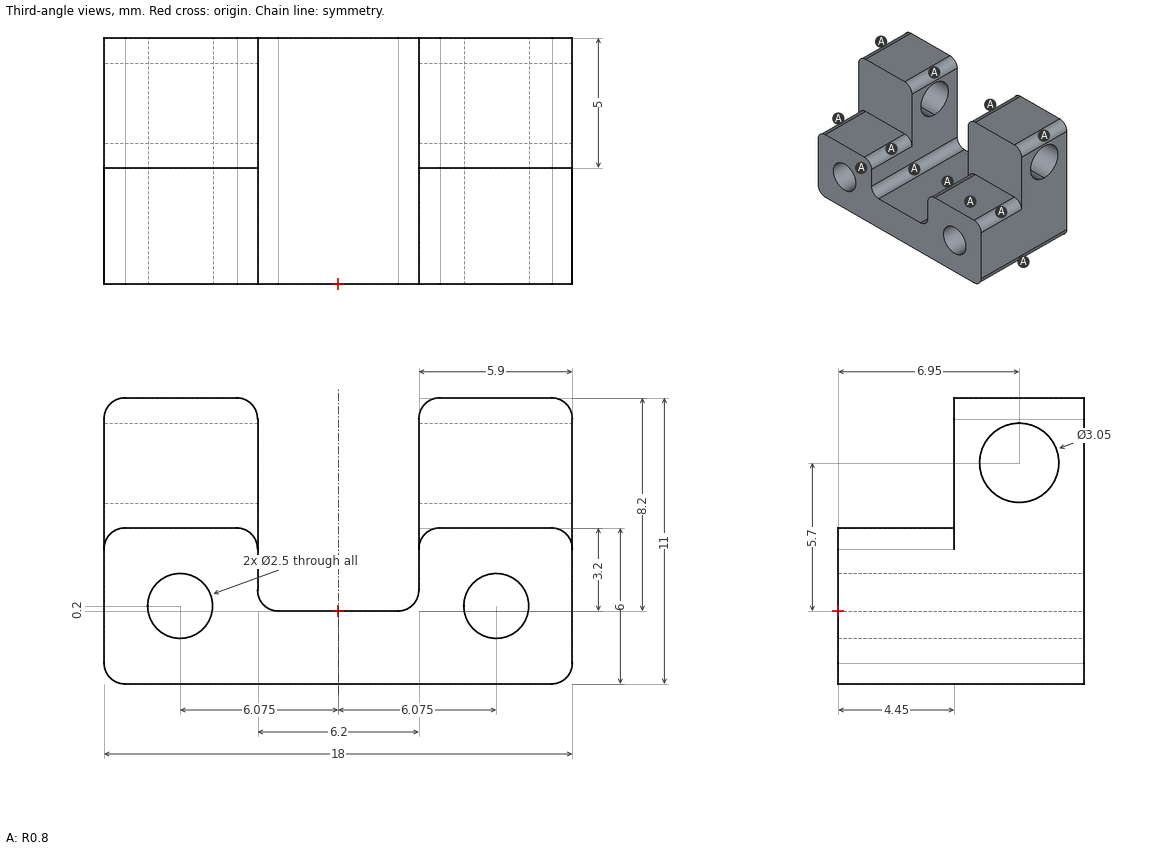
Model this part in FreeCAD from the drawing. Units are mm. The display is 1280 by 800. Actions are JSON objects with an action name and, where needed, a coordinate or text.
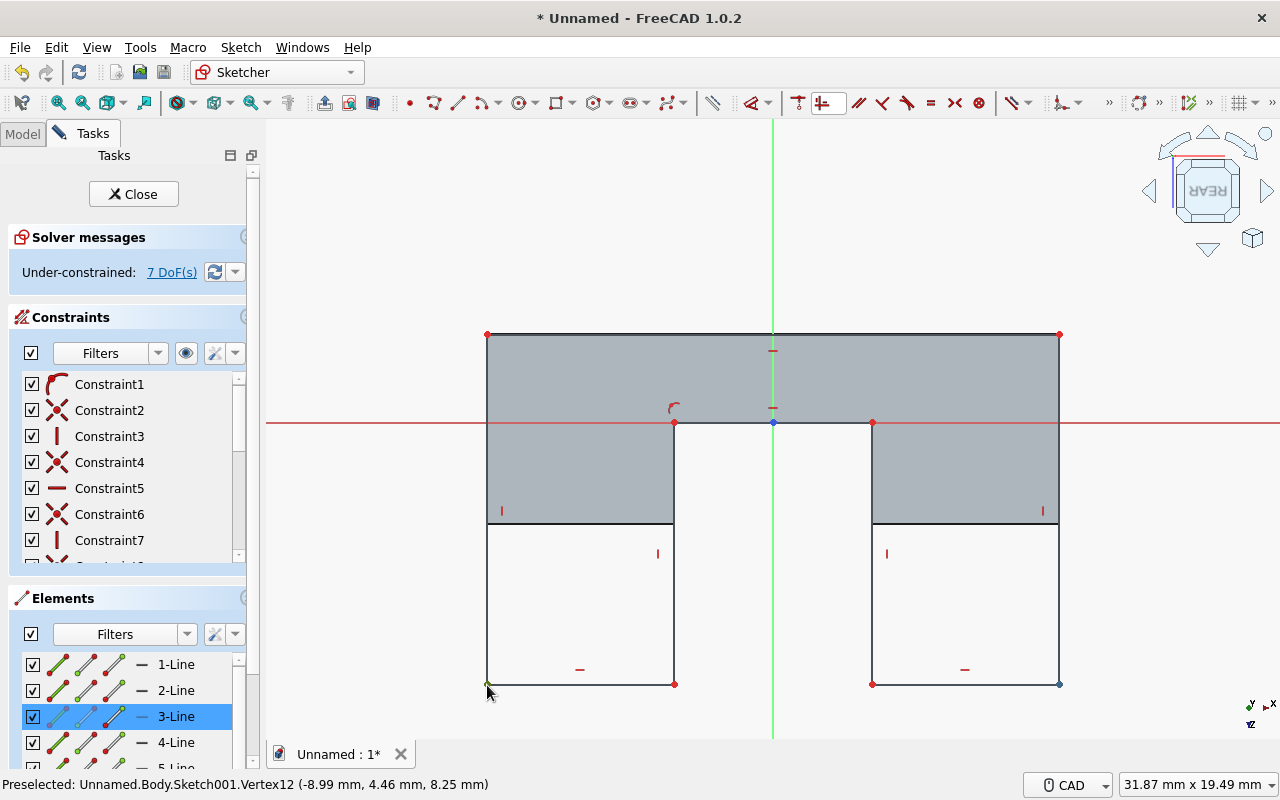
{"action": "left_click", "coordinate": [773, 671]}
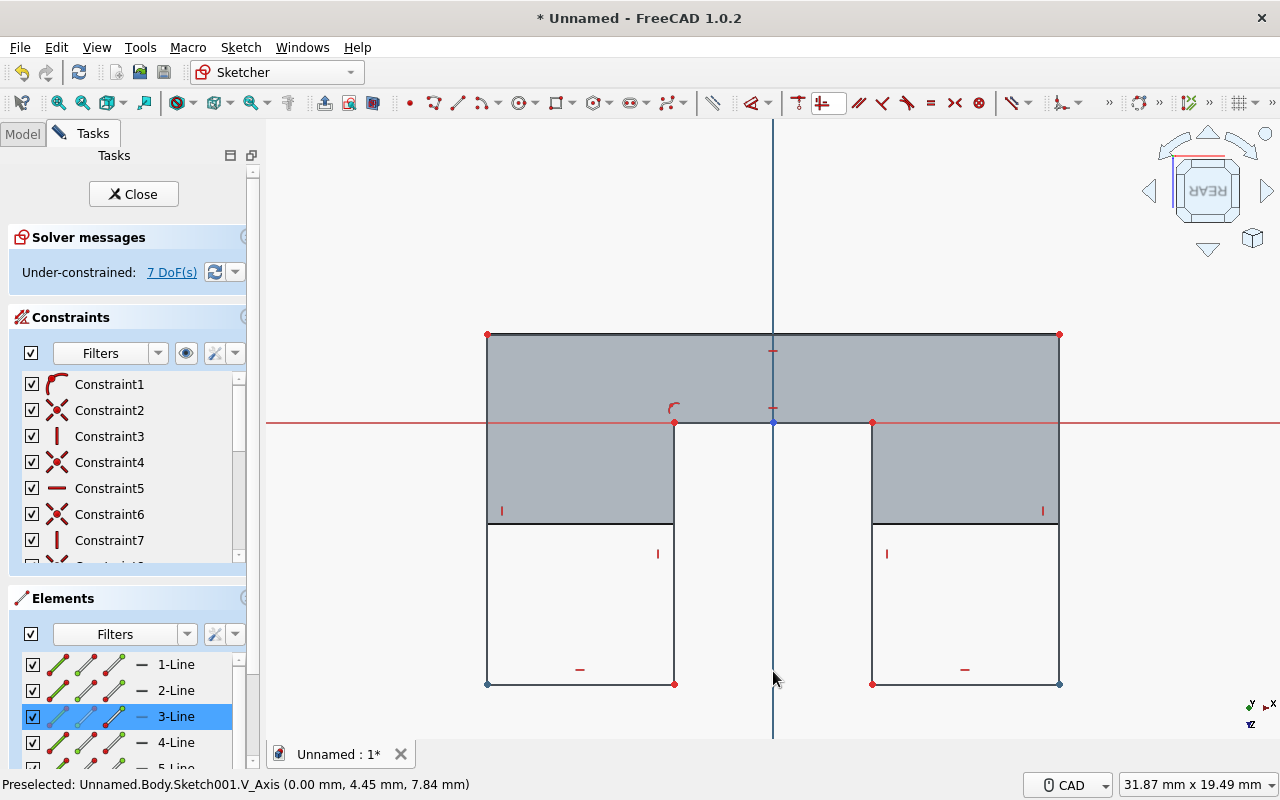
{"action": "left_click", "coordinate": [956, 104]}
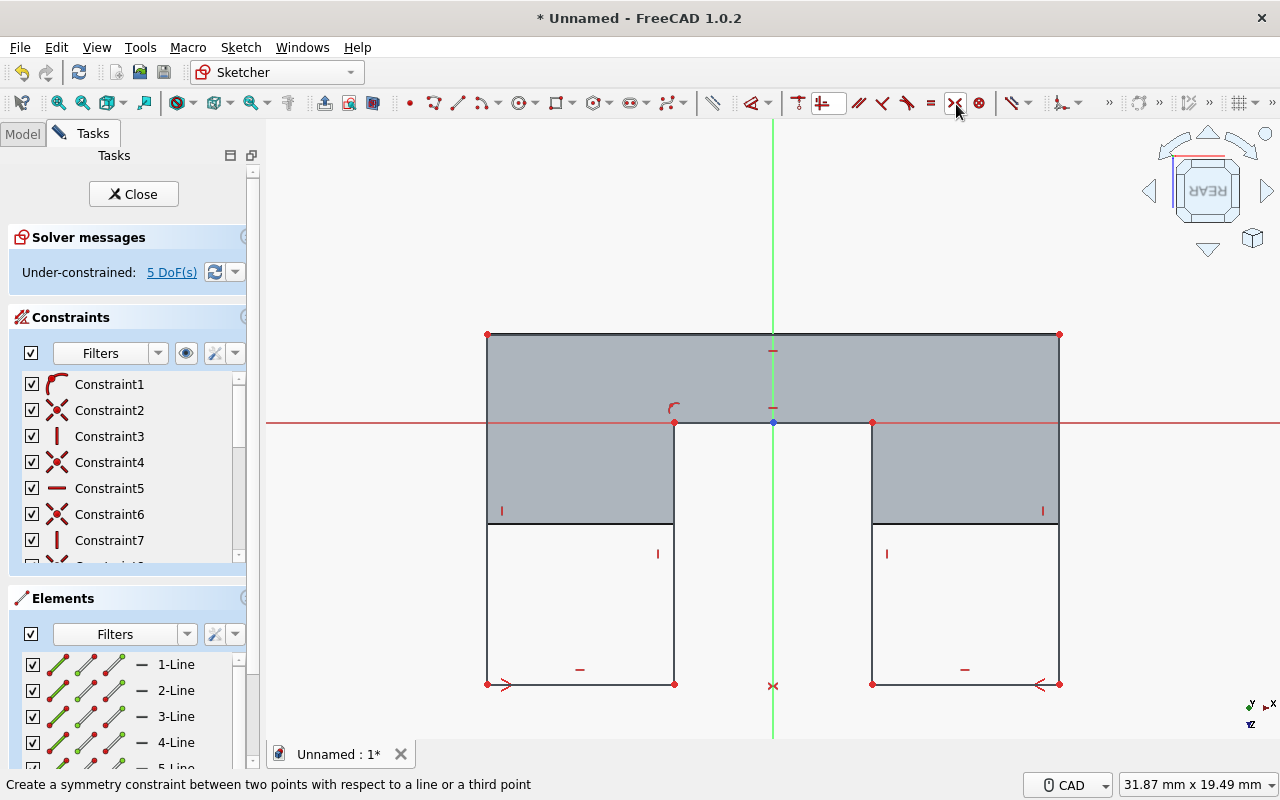
{"action": "left_click", "coordinate": [752, 104]}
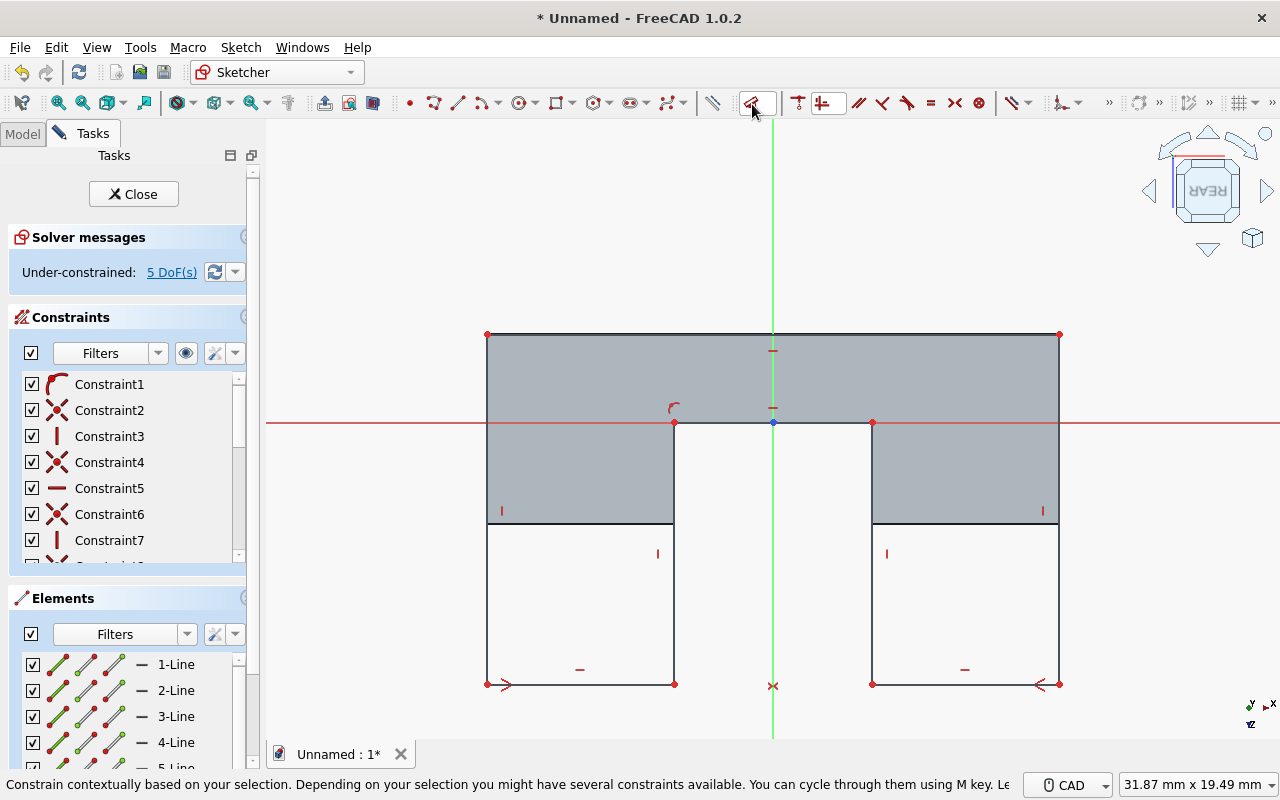
{"action": "left_click", "coordinate": [1059, 580]}
{"action": "left_click", "coordinate": [1093, 510]}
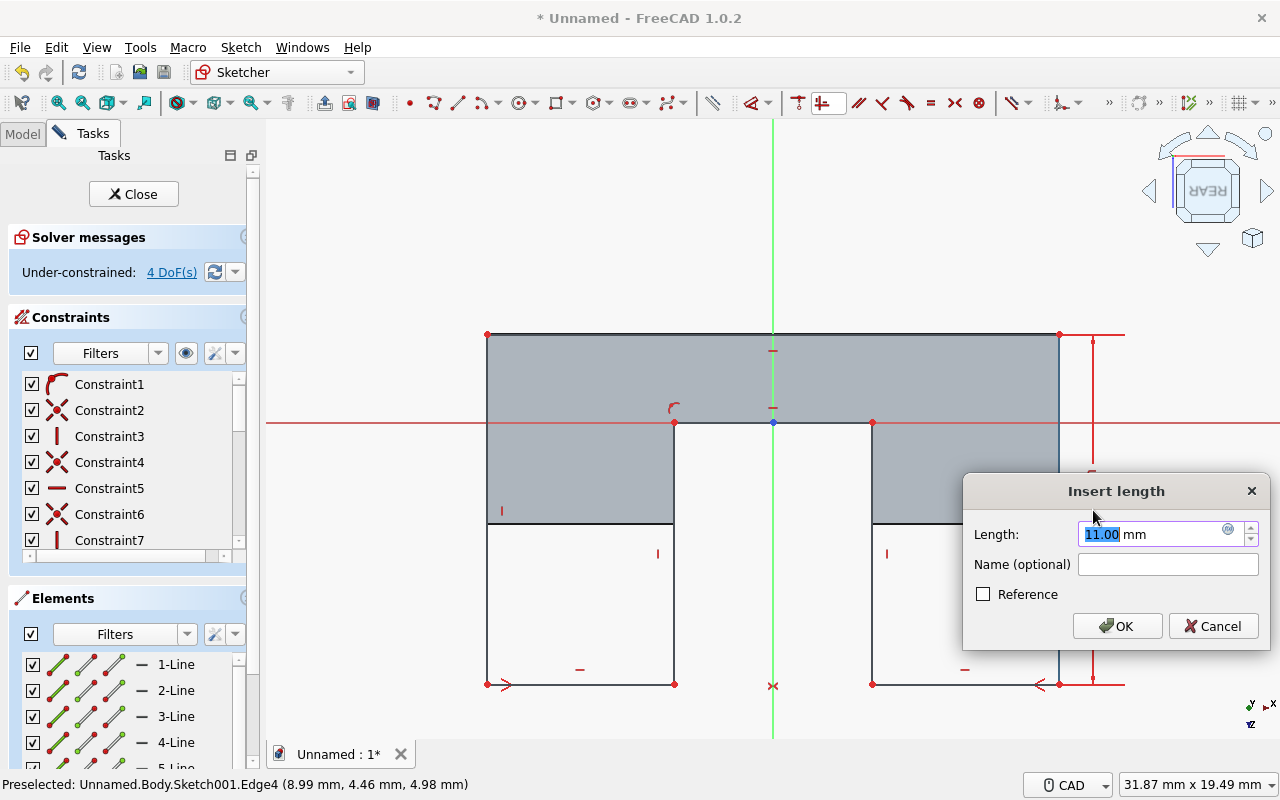
{"action": "type", "text": "11"}
{"action": "key", "text": "Return"}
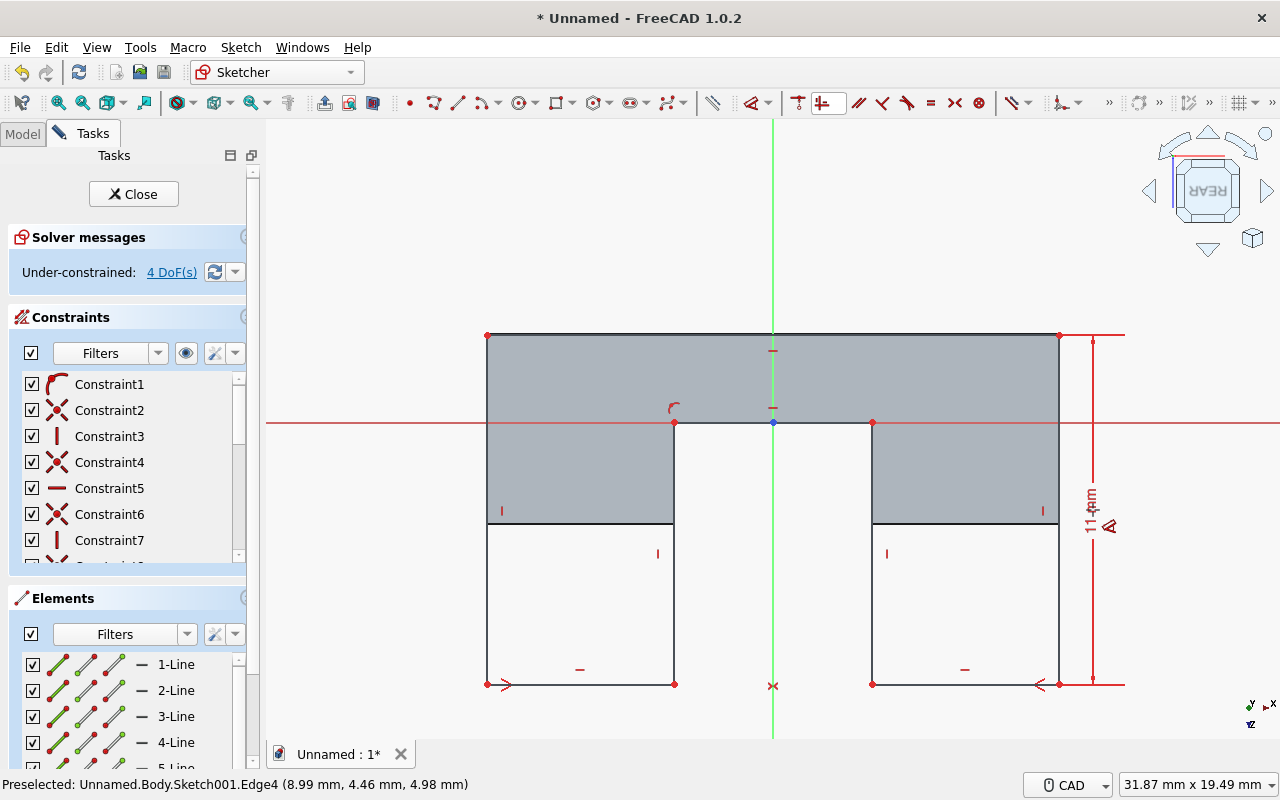
{"action": "left_click", "coordinate": [887, 335]}
{"action": "left_click", "coordinate": [641, 301]}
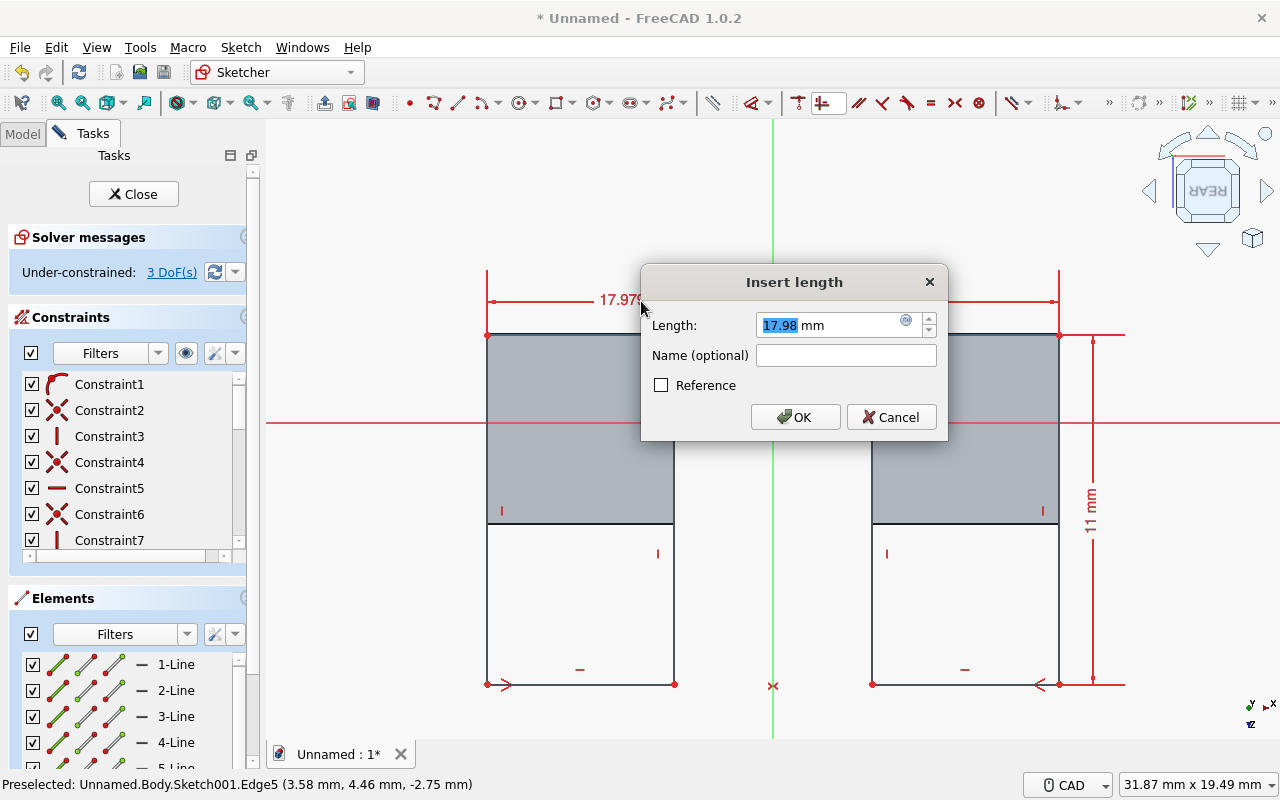
{"action": "type", "text": "18"}
{"action": "key", "text": "Return"}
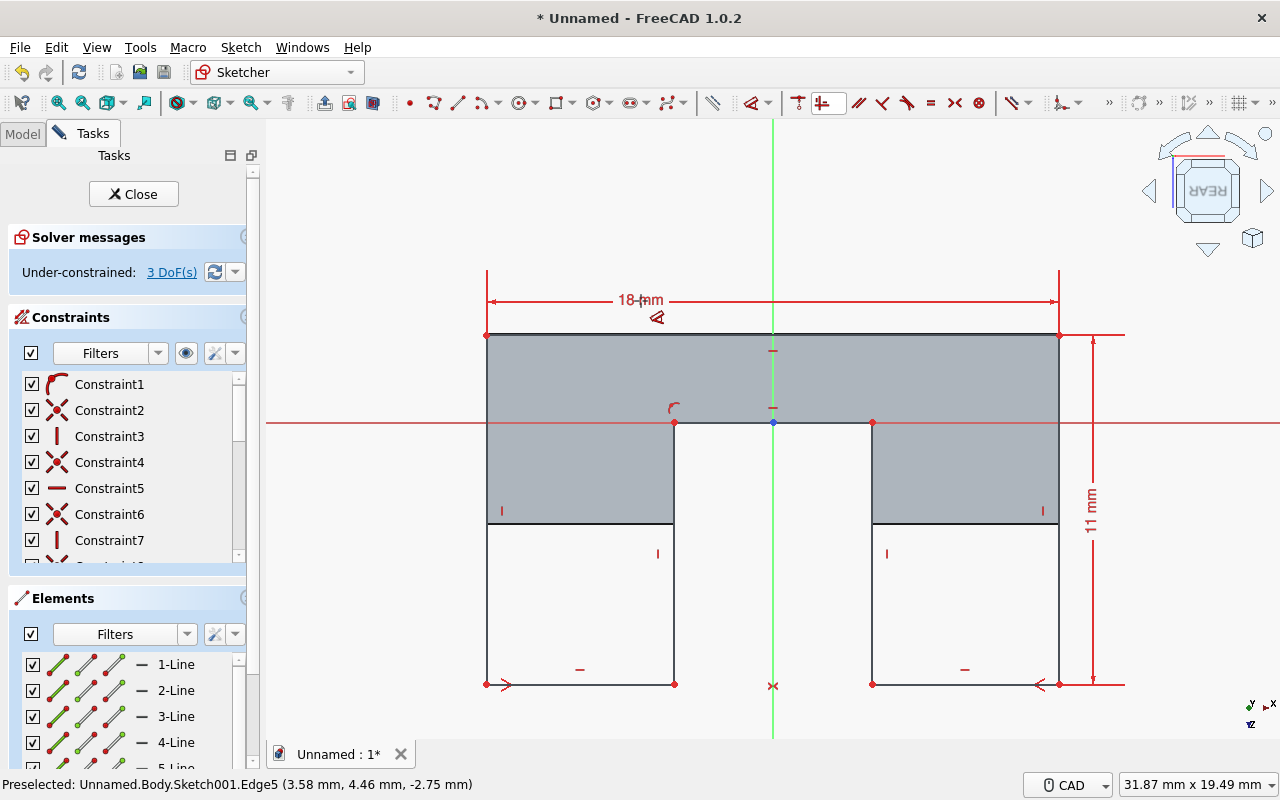
{"action": "left_click", "coordinate": [733, 423]}
{"action": "left_click", "coordinate": [727, 389]}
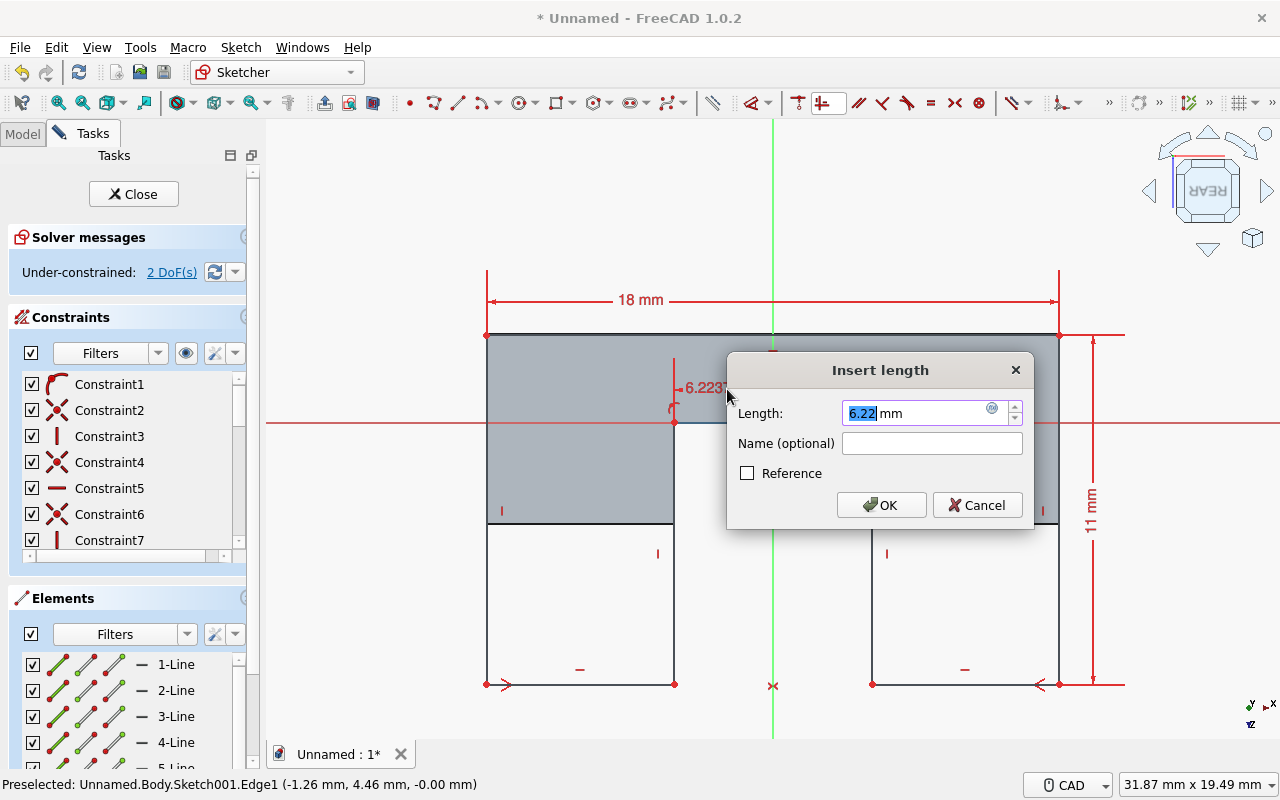
{"action": "type", "text": "6.2"}
{"action": "key", "text": "Return"}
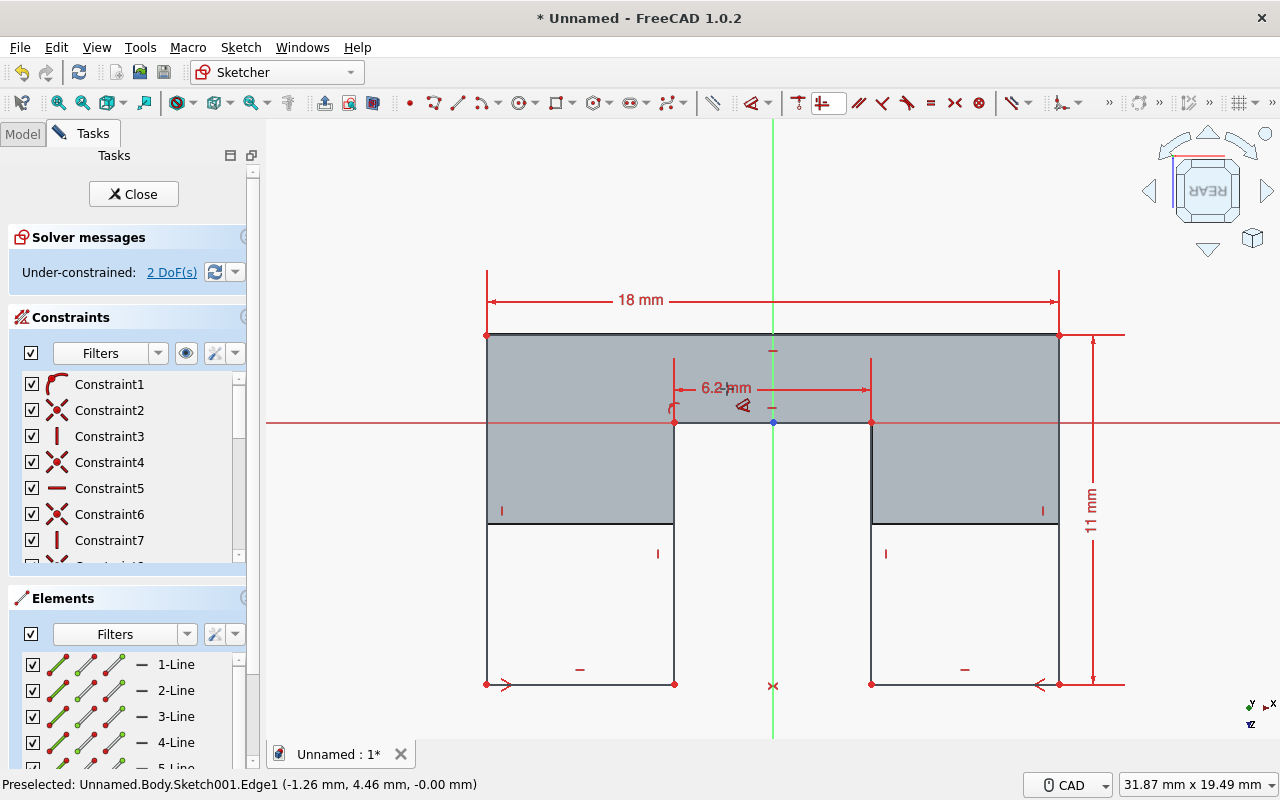
{"action": "left_click", "coordinate": [871, 501]}
{"action": "left_click", "coordinate": [905, 554]}